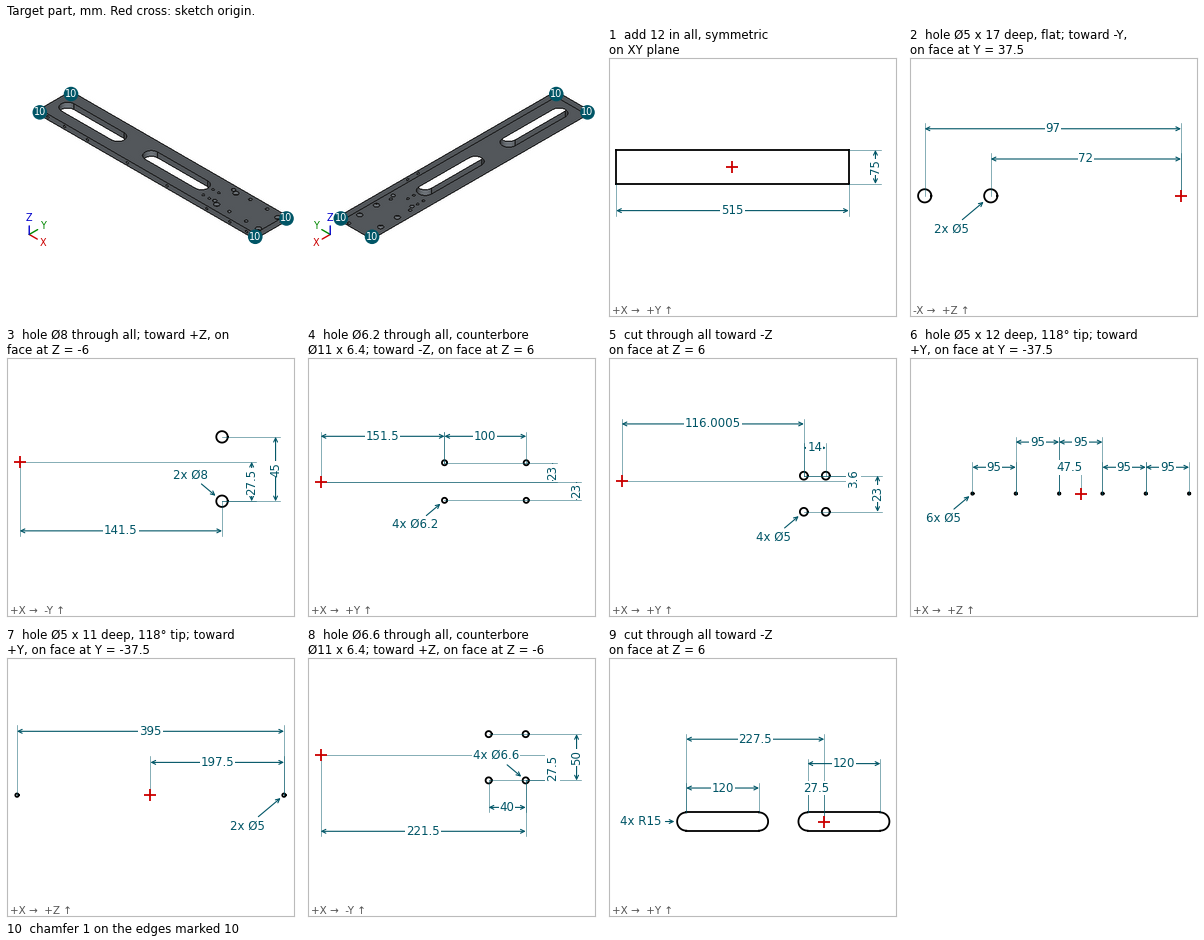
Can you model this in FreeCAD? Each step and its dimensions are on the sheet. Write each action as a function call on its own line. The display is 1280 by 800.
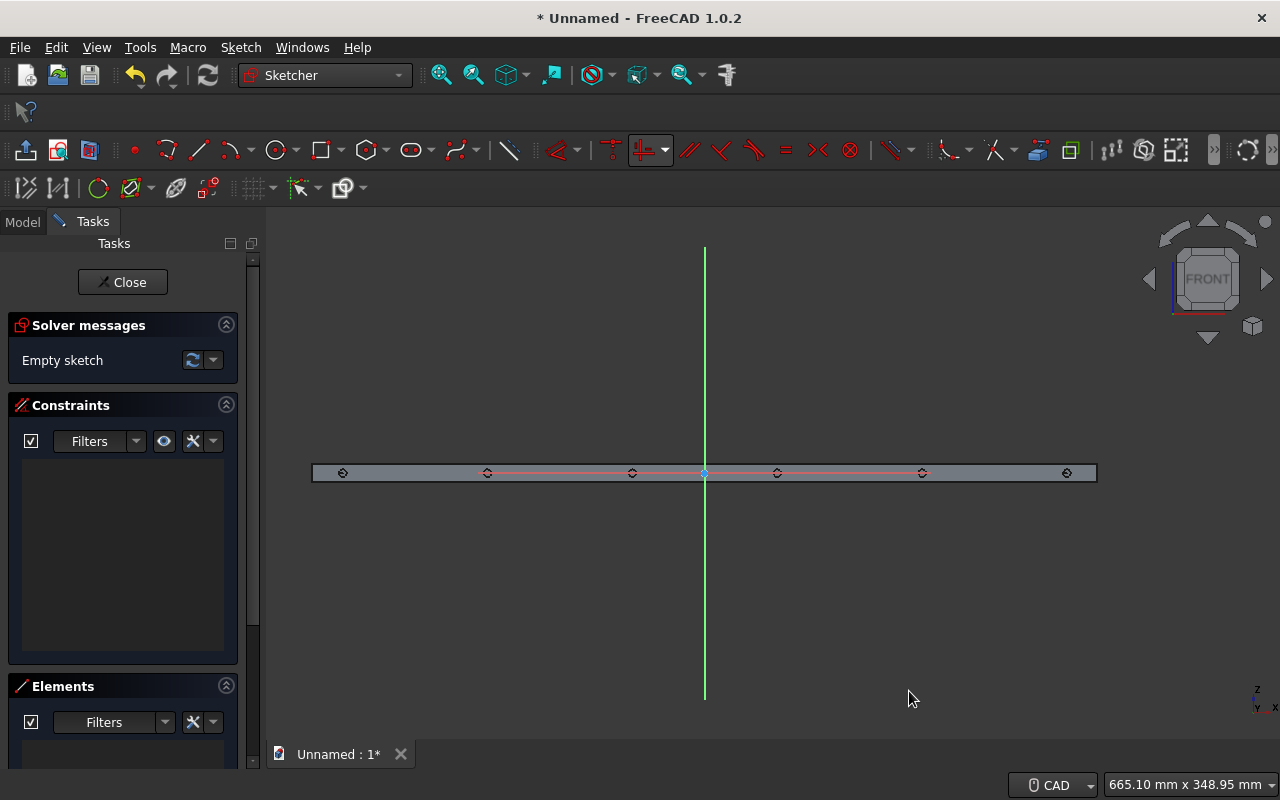
key(g)
key(c)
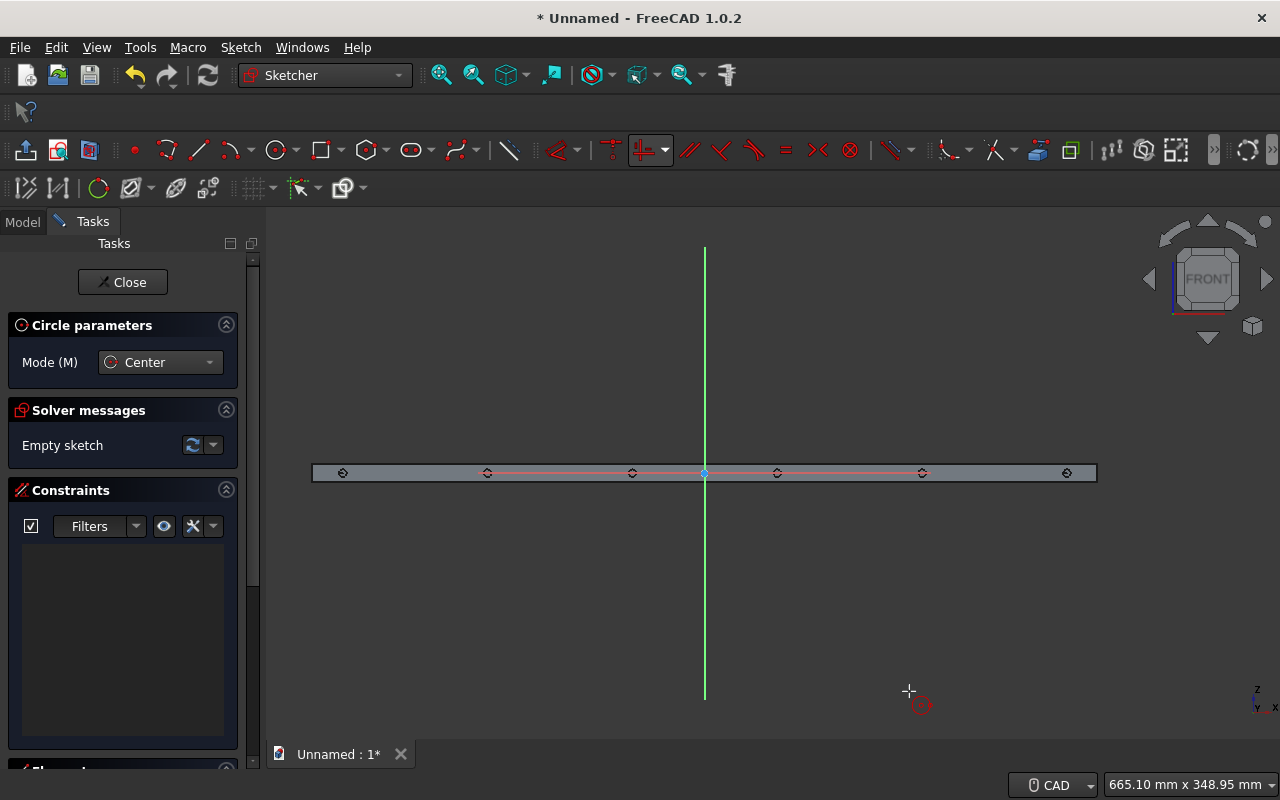
scroll(1006, 473, up, 9)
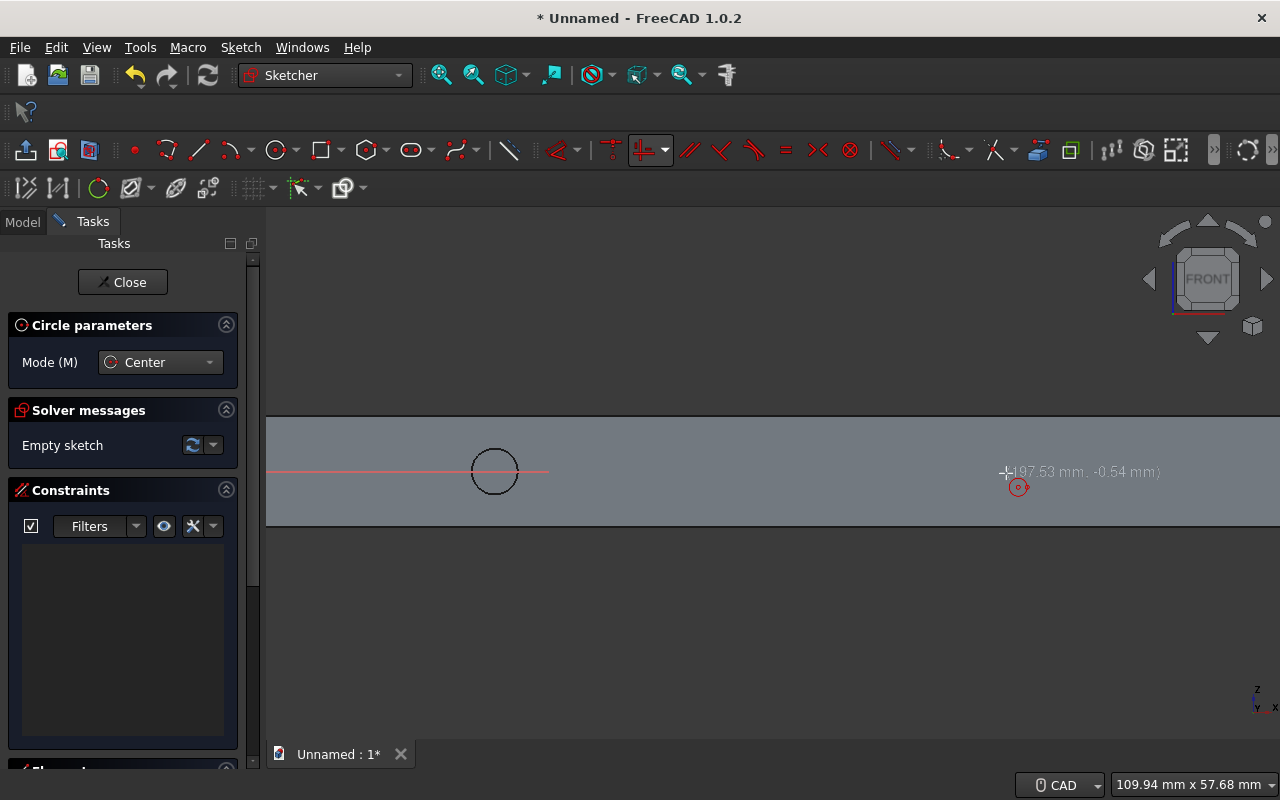
scroll(1006, 473, down, 9)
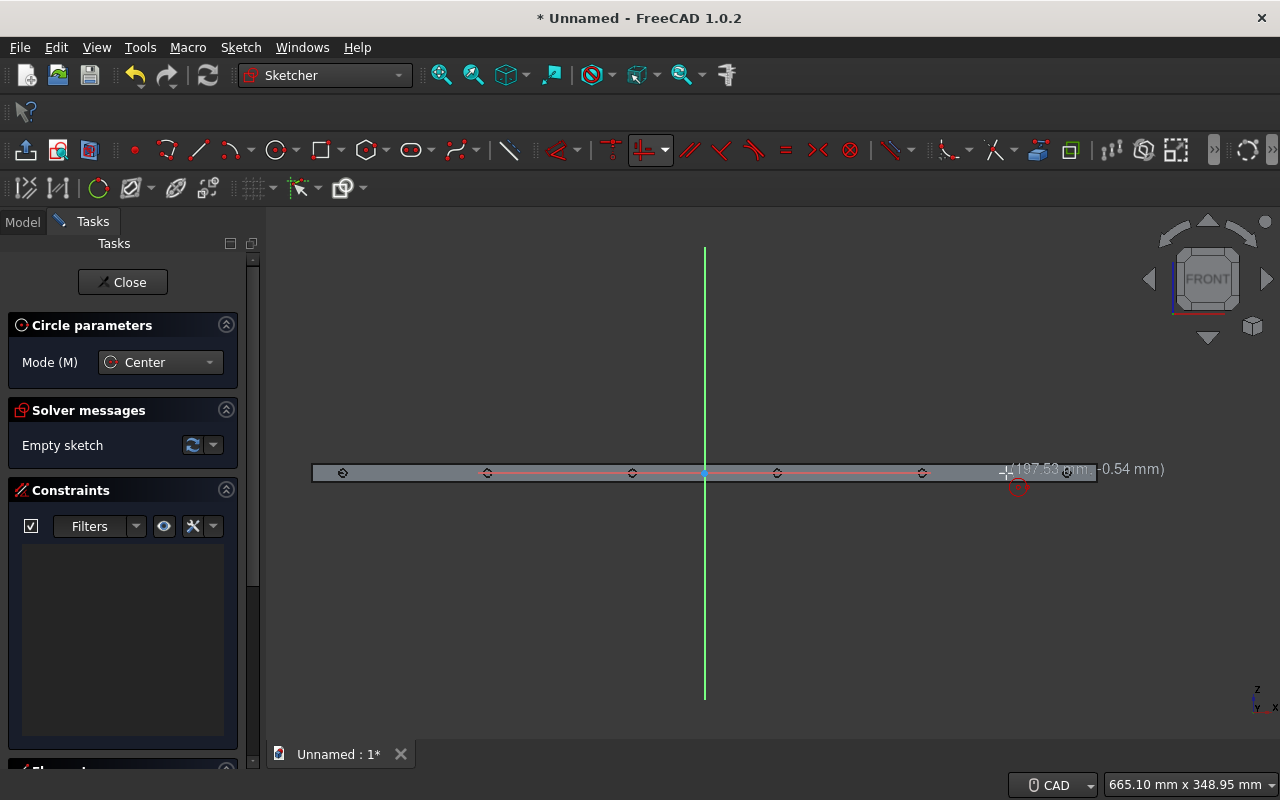
click(1006, 473)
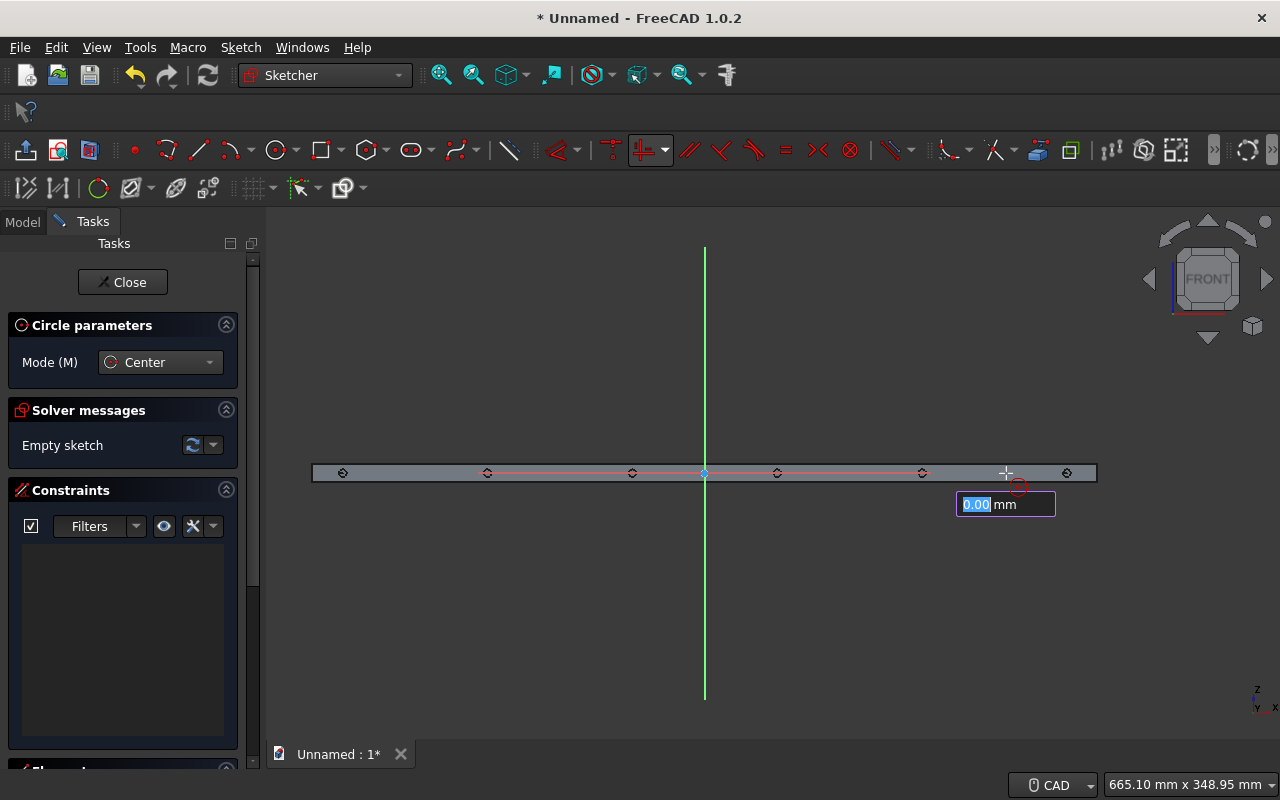
scroll(1005, 477, up, 8)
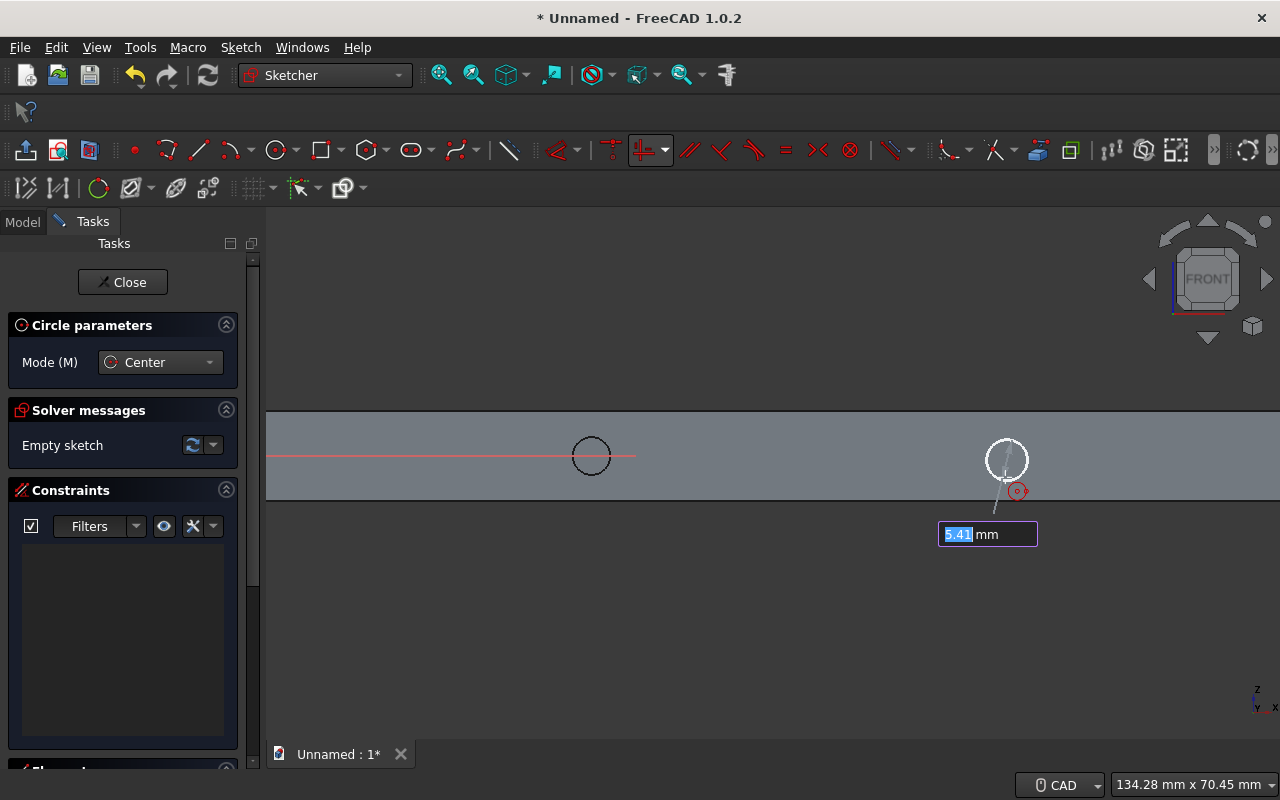
click(1000, 474)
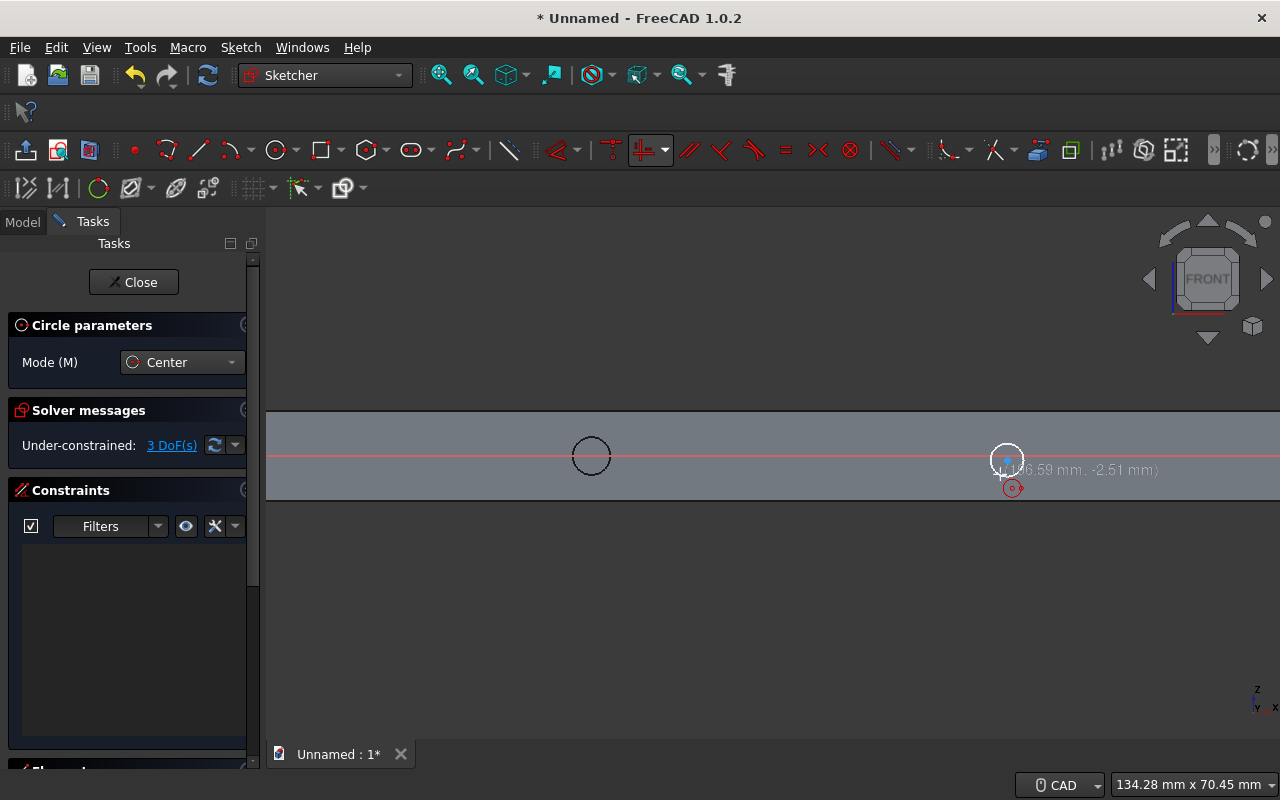
scroll(1005, 477, down, 8)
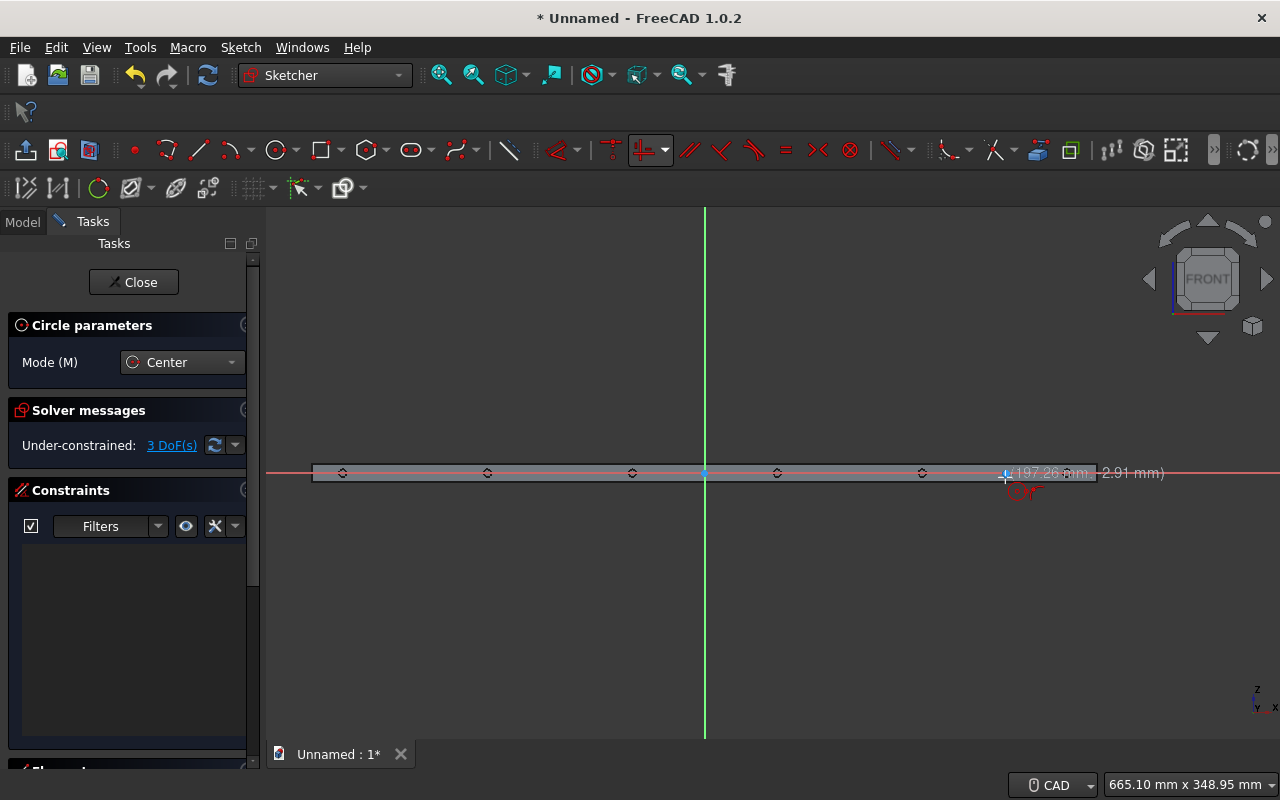
scroll(404, 473, up, 9)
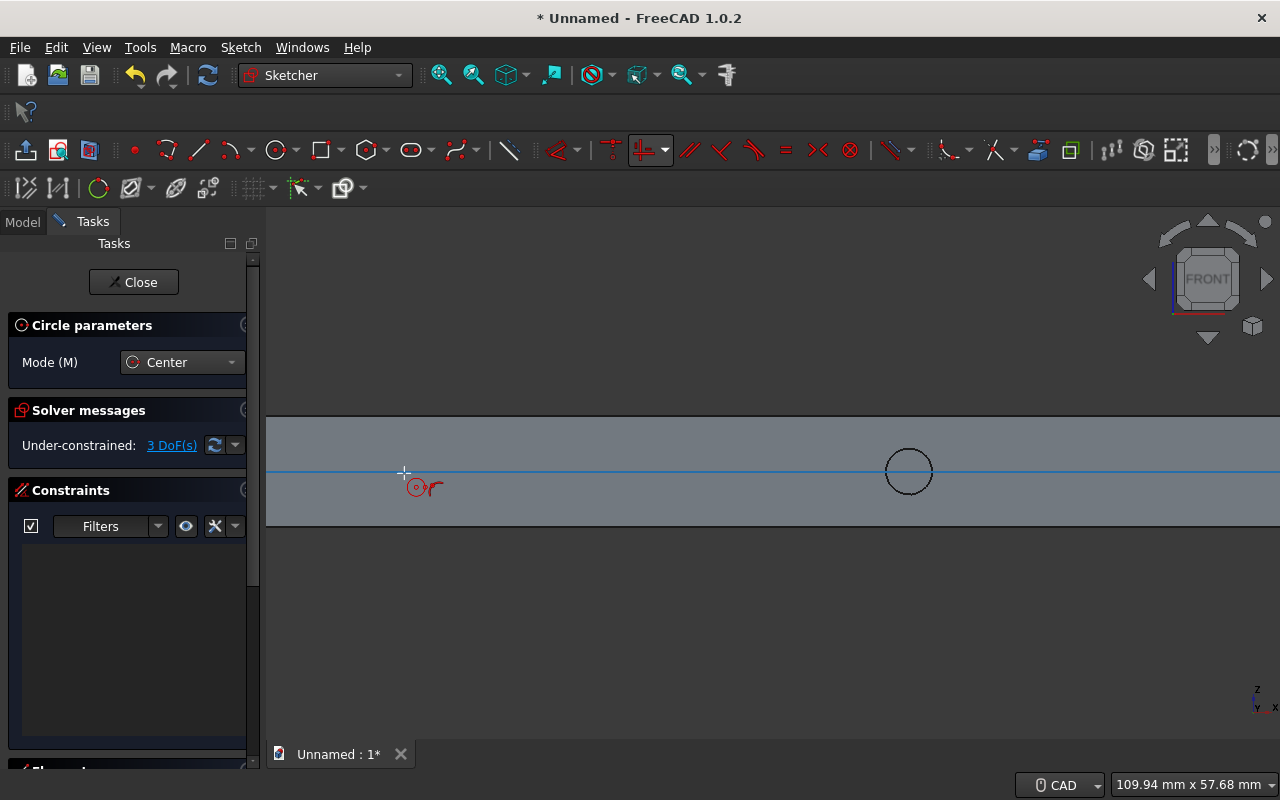
scroll(404, 473, down, 9)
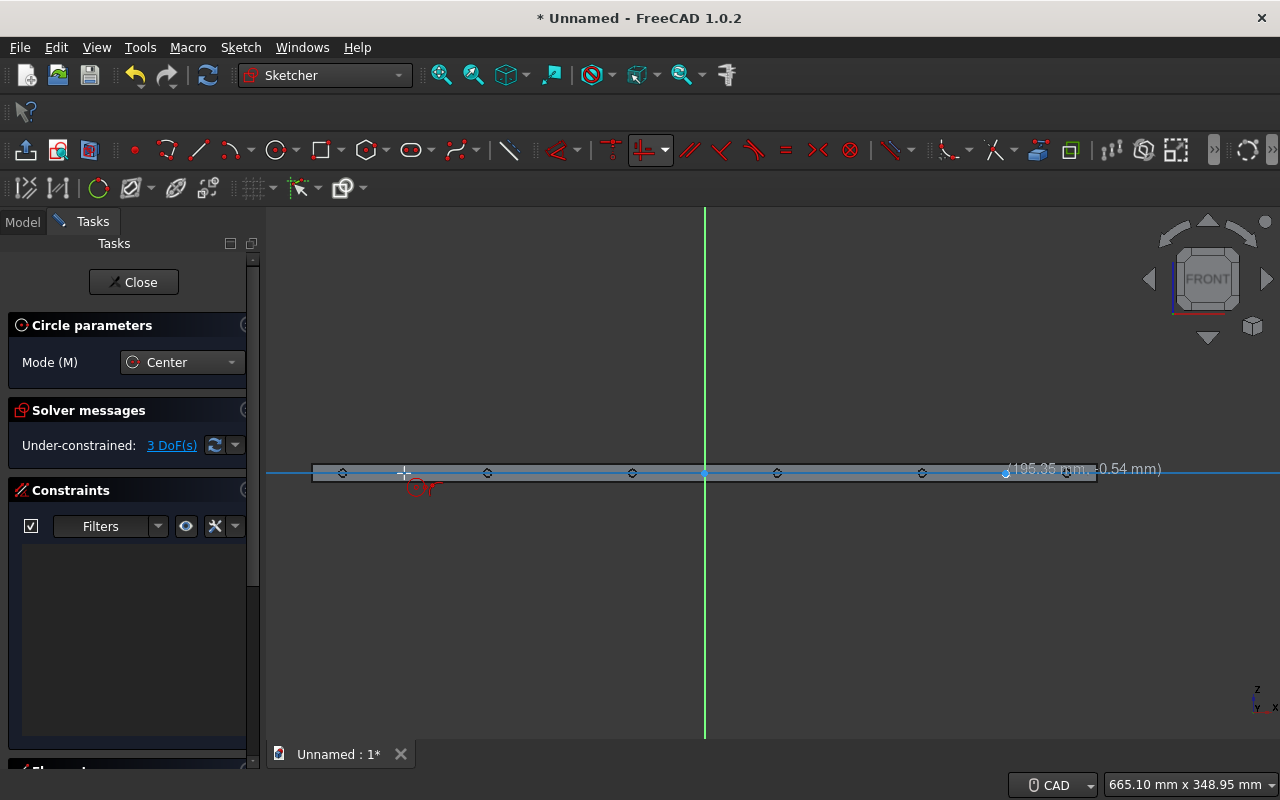
click(404, 473)